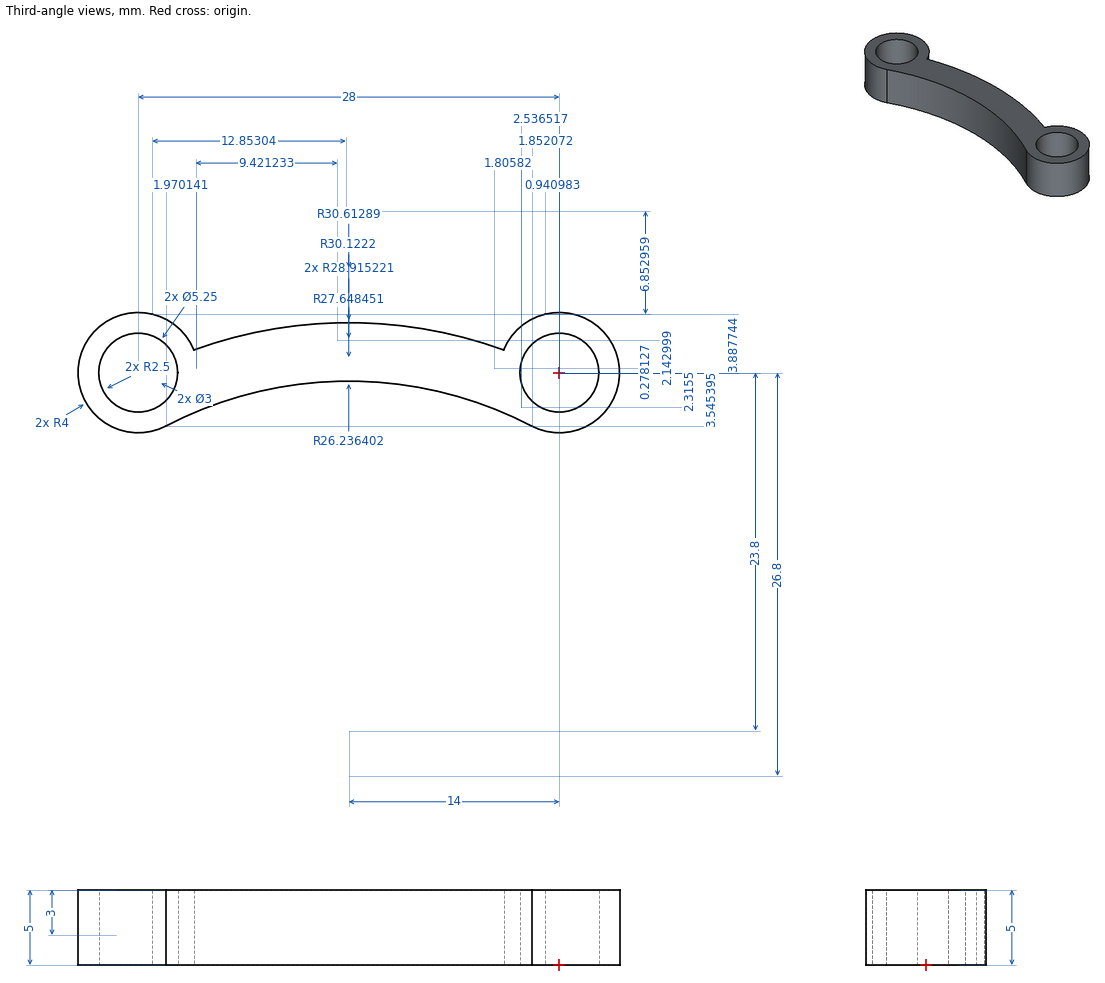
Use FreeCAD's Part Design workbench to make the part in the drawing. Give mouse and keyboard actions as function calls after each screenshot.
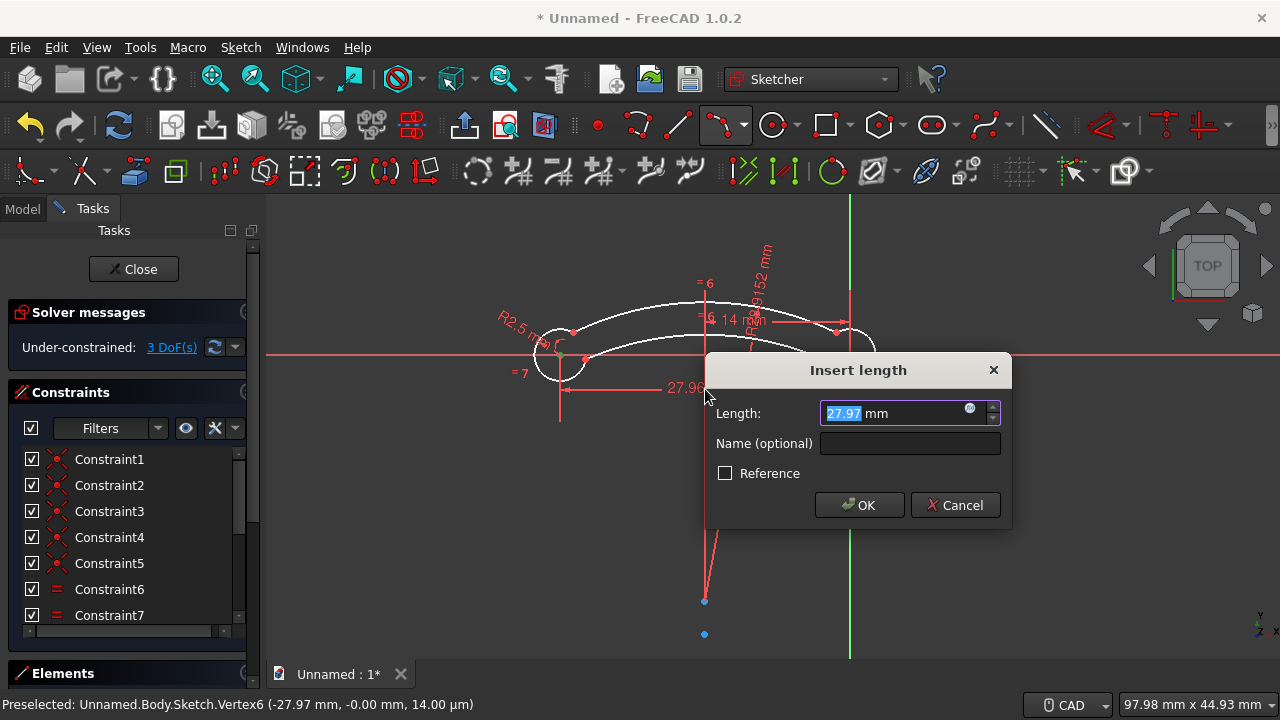
text(28)
key(Return)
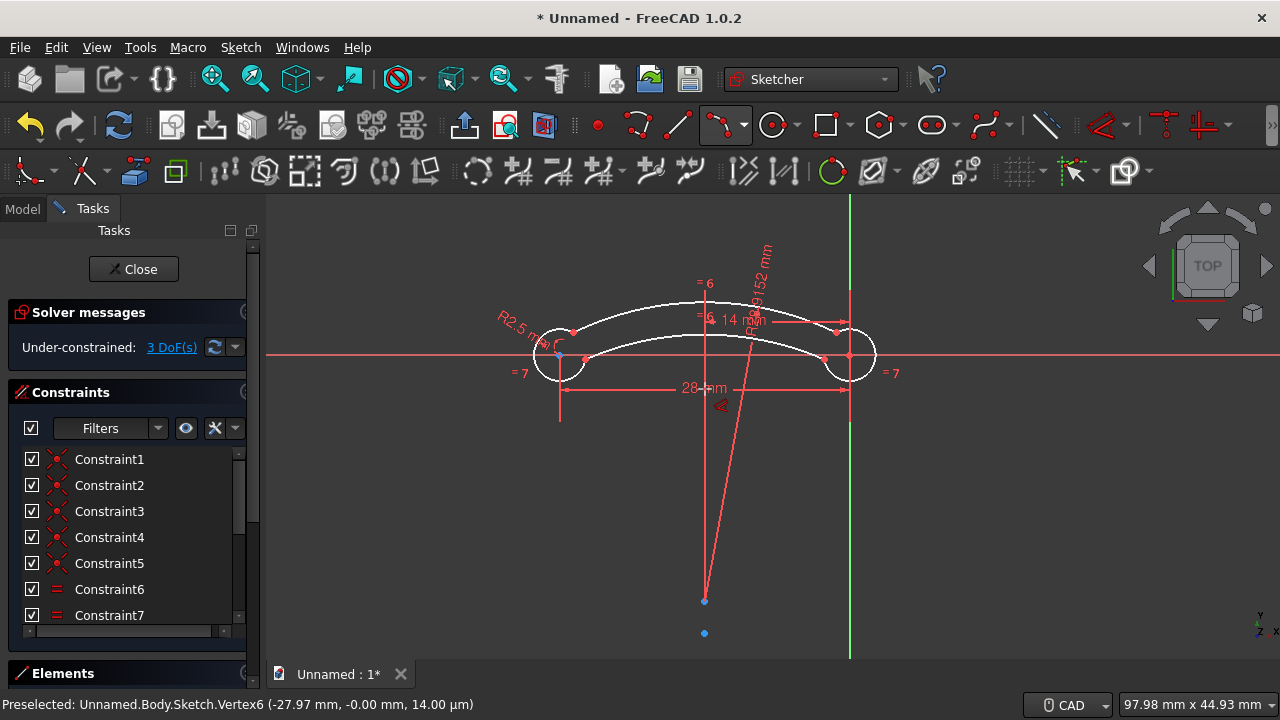
scroll(705, 222, up, 3)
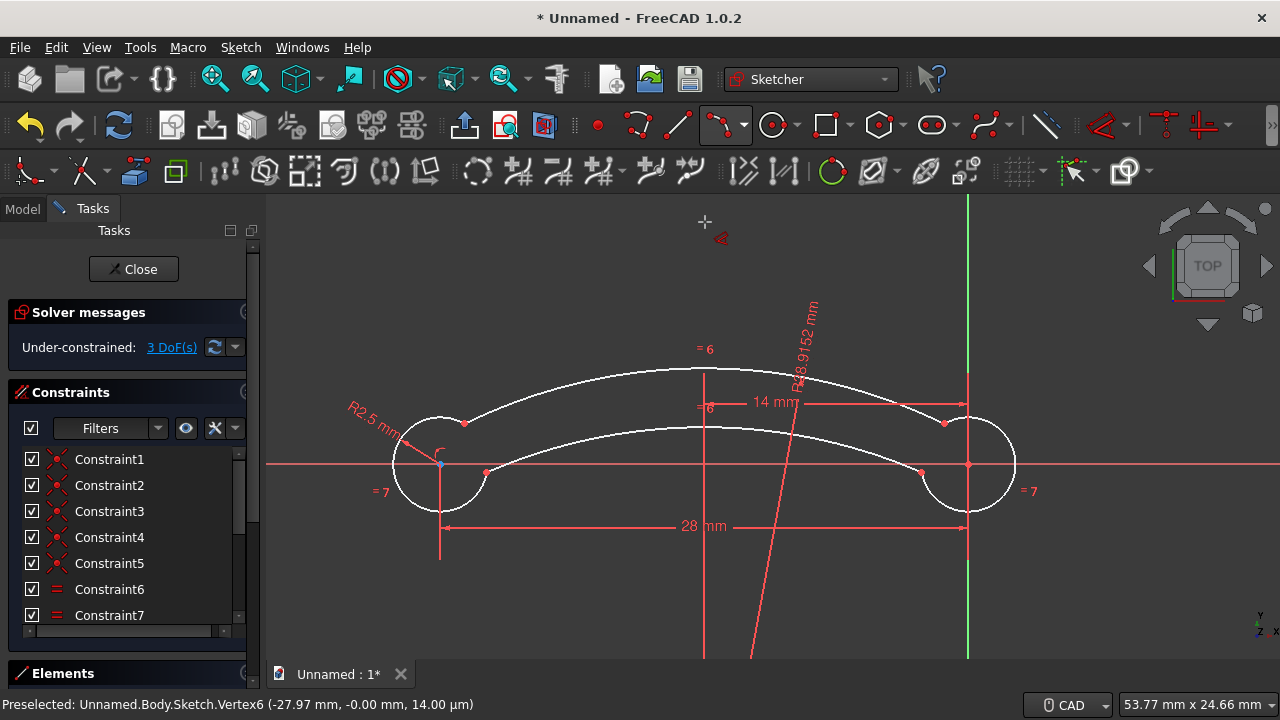
scroll(705, 228, down, 4)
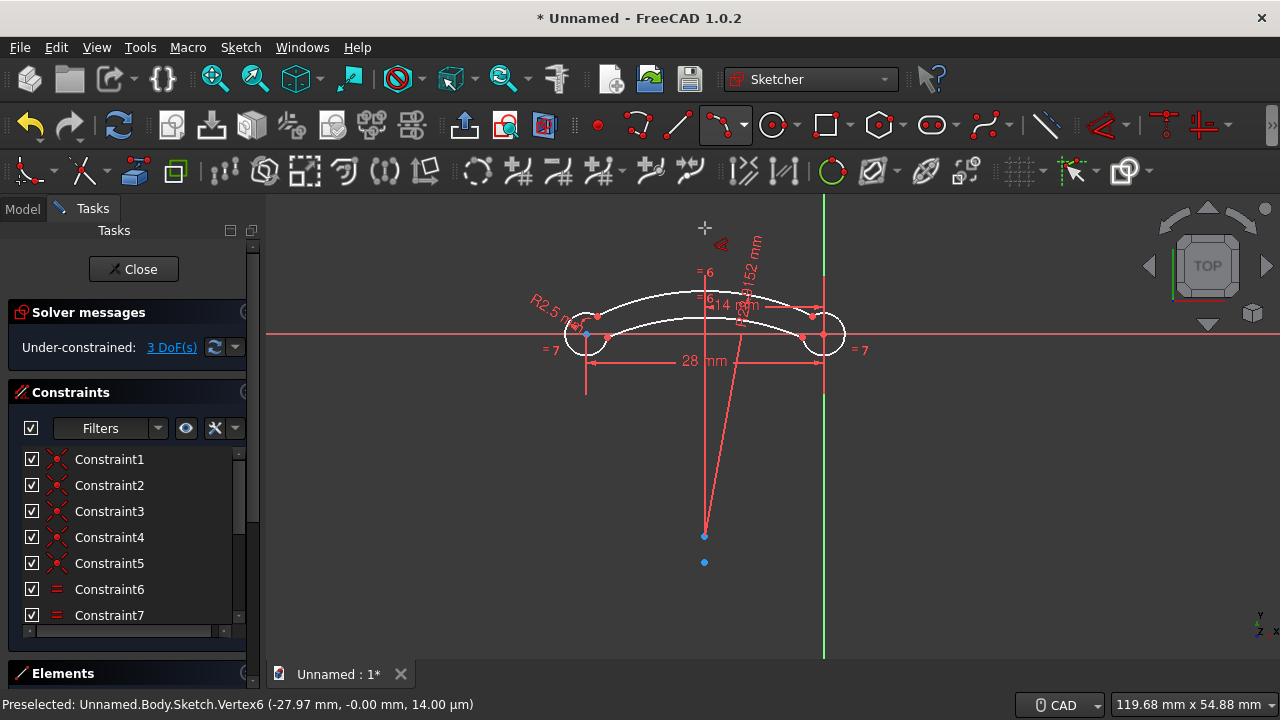
click(705, 563)
click(764, 597)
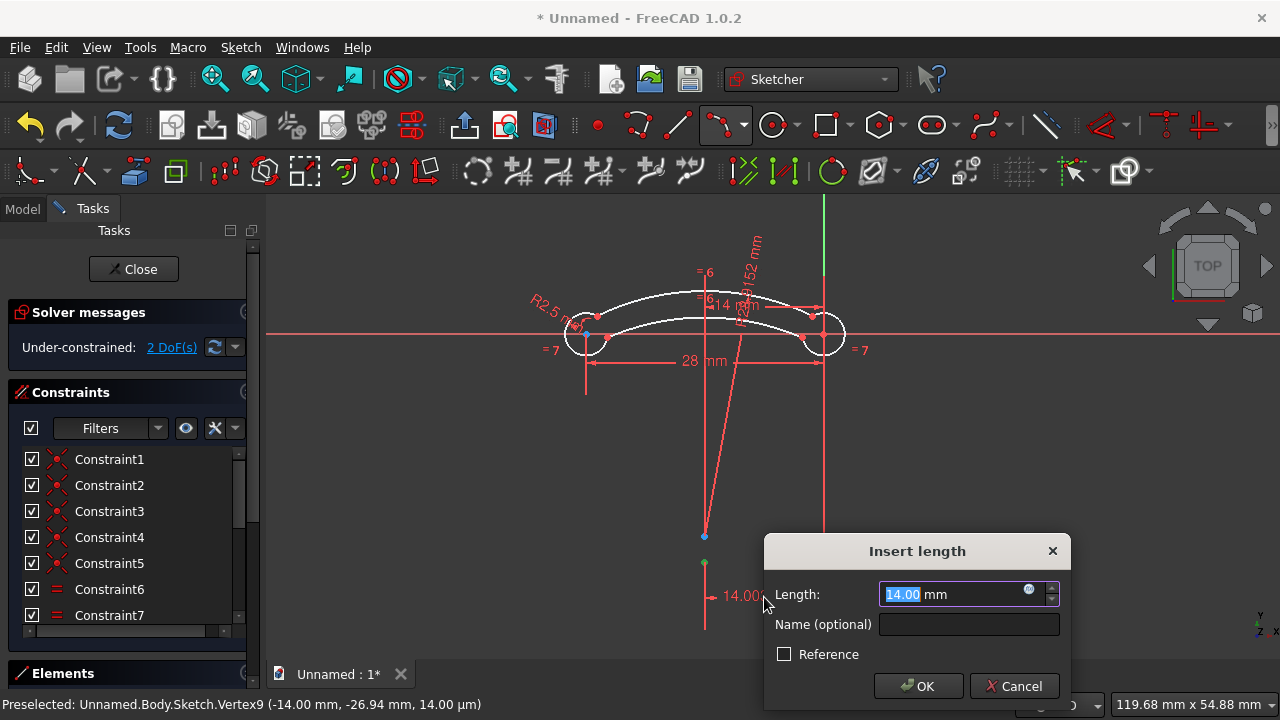
text(14)
key(Return)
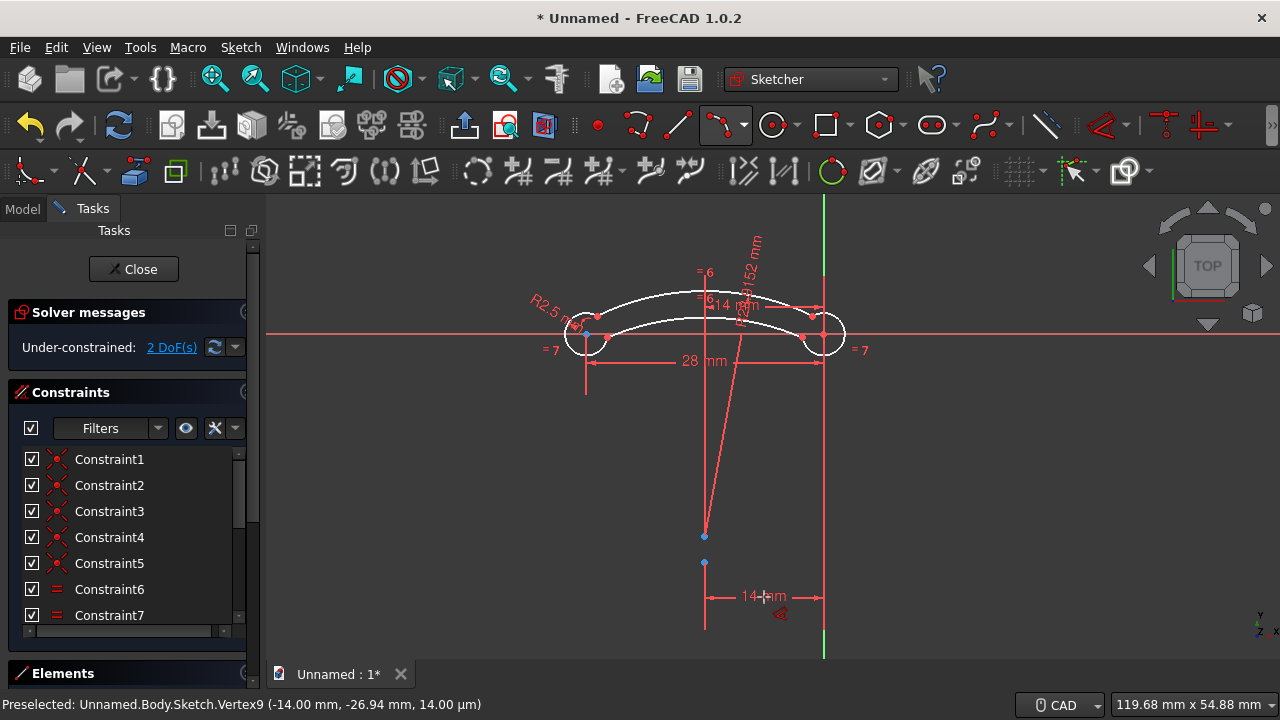
click(705, 536)
click(858, 435)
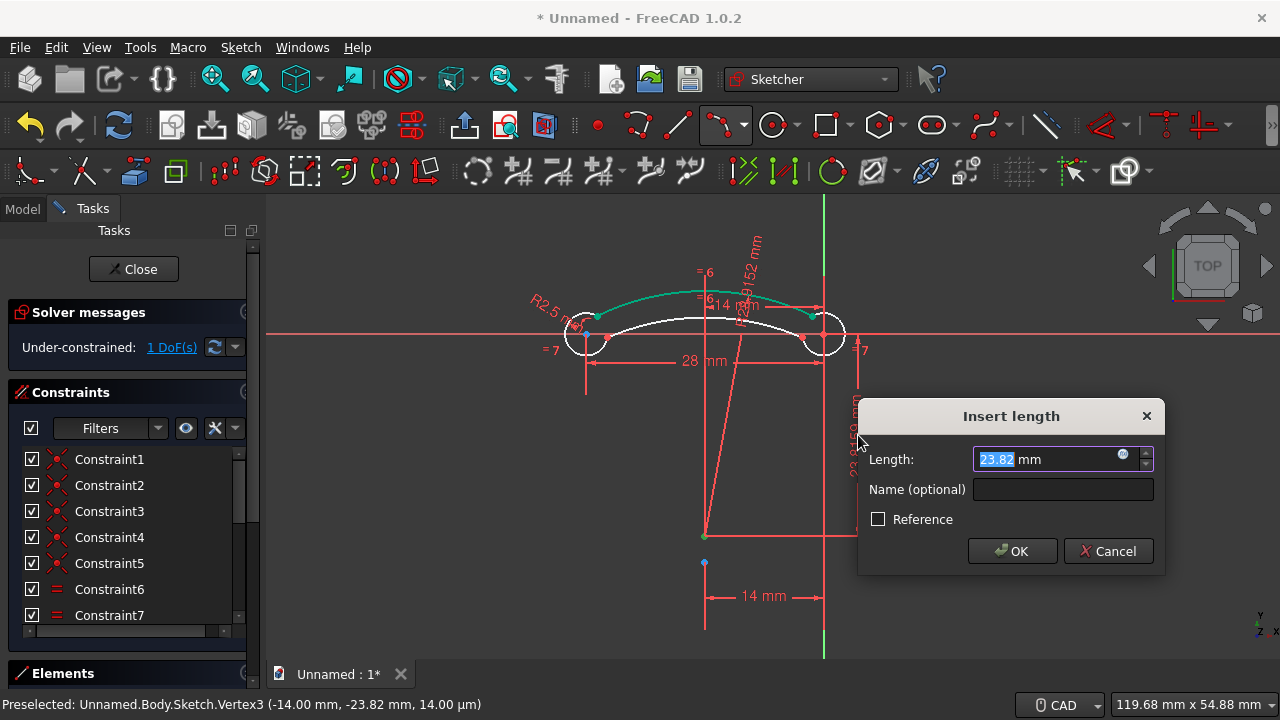
text(23.8)
key(Return)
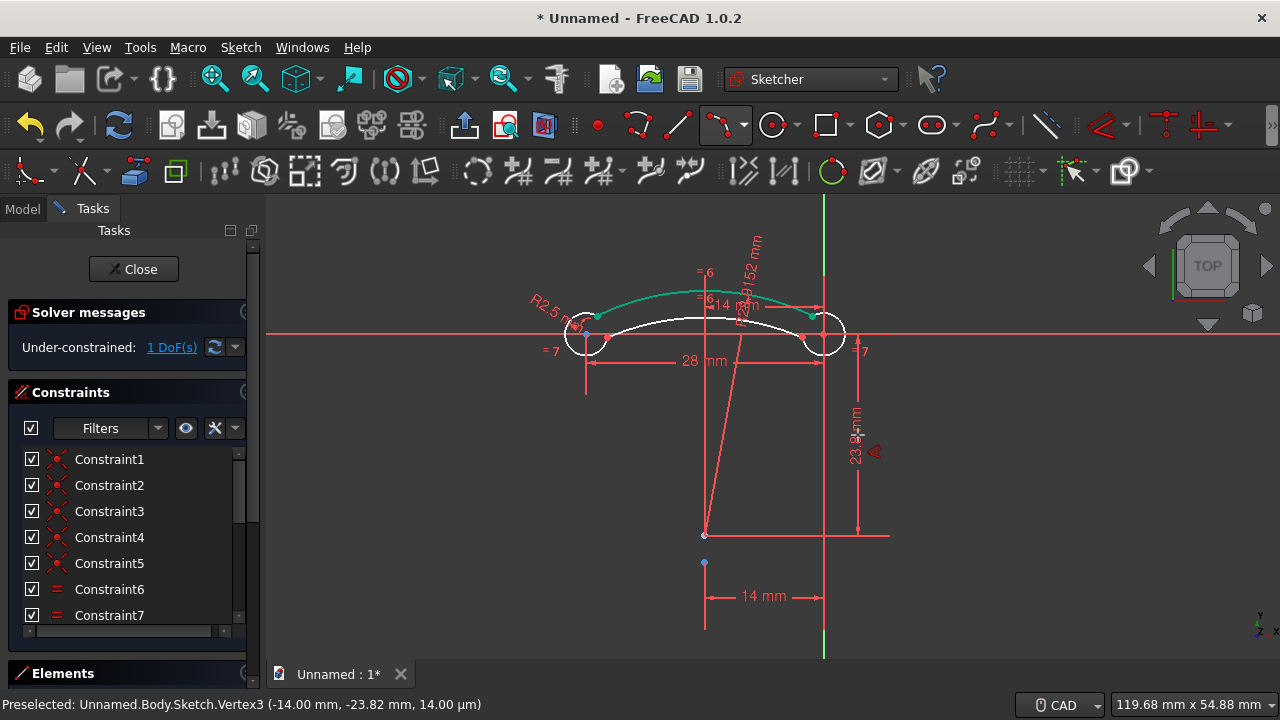
click(705, 563)
click(858, 396)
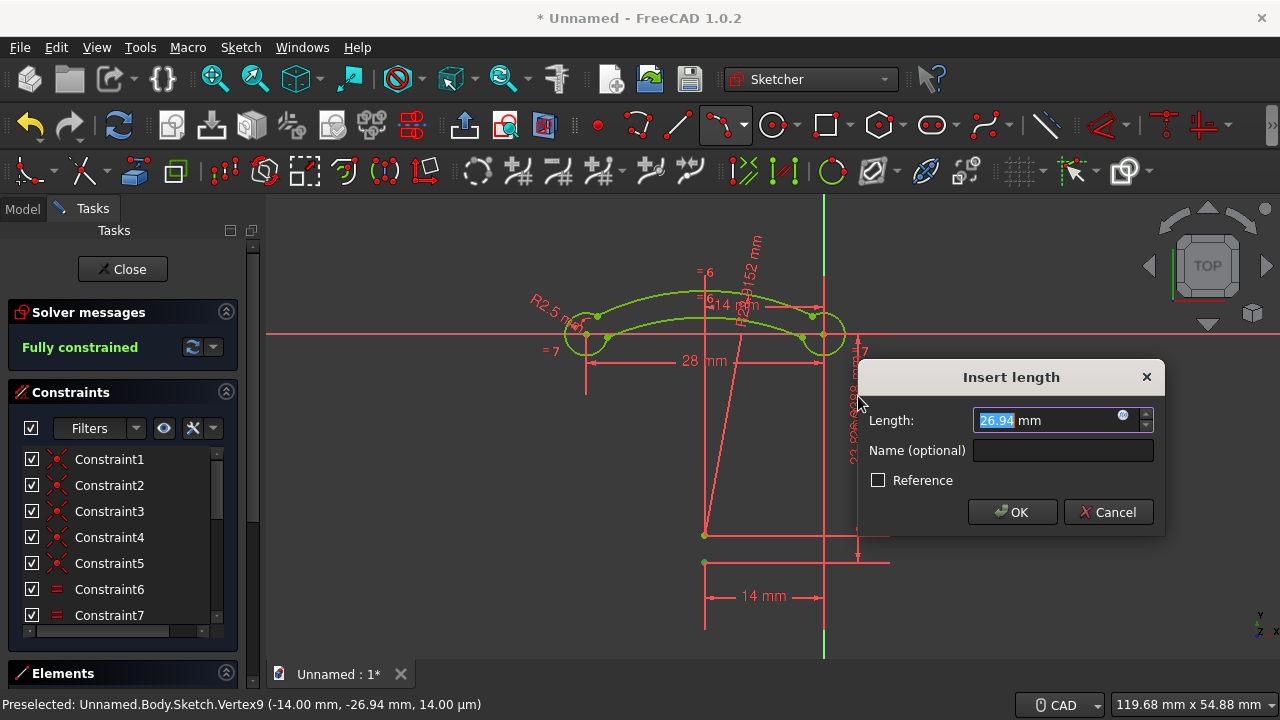
text(26.8)
key(Return)
key(Escape)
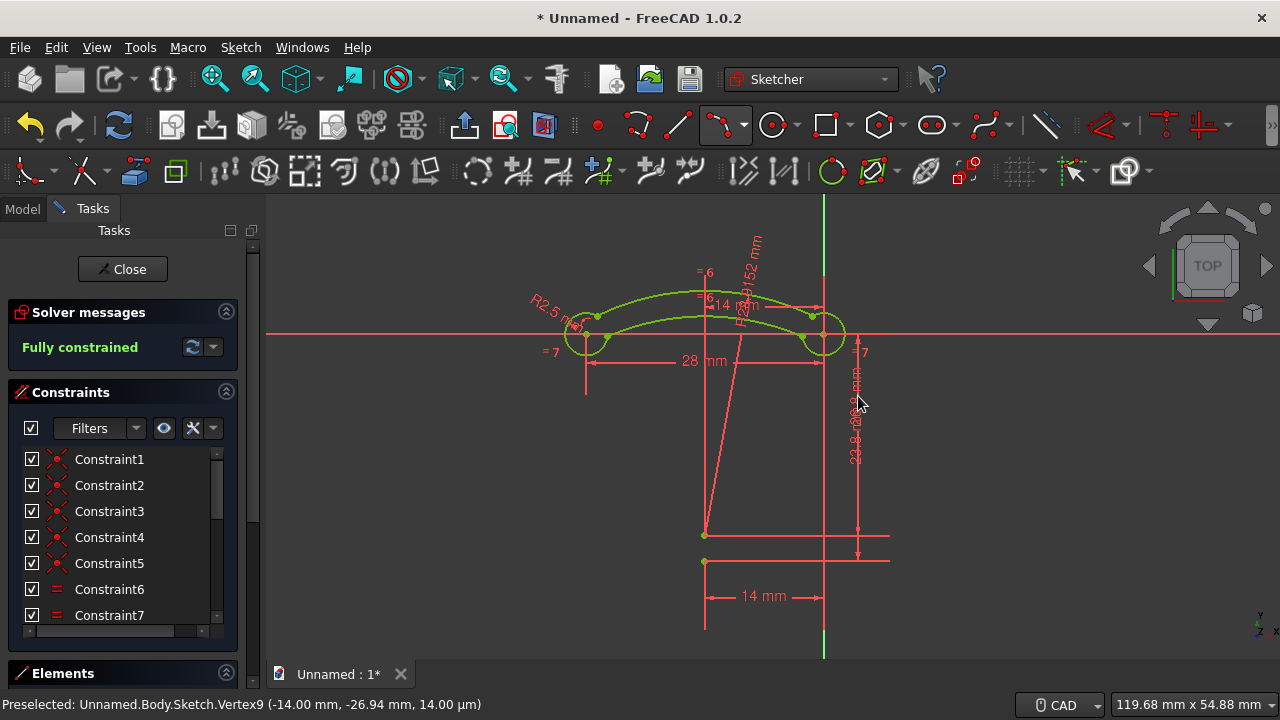
click(123, 269)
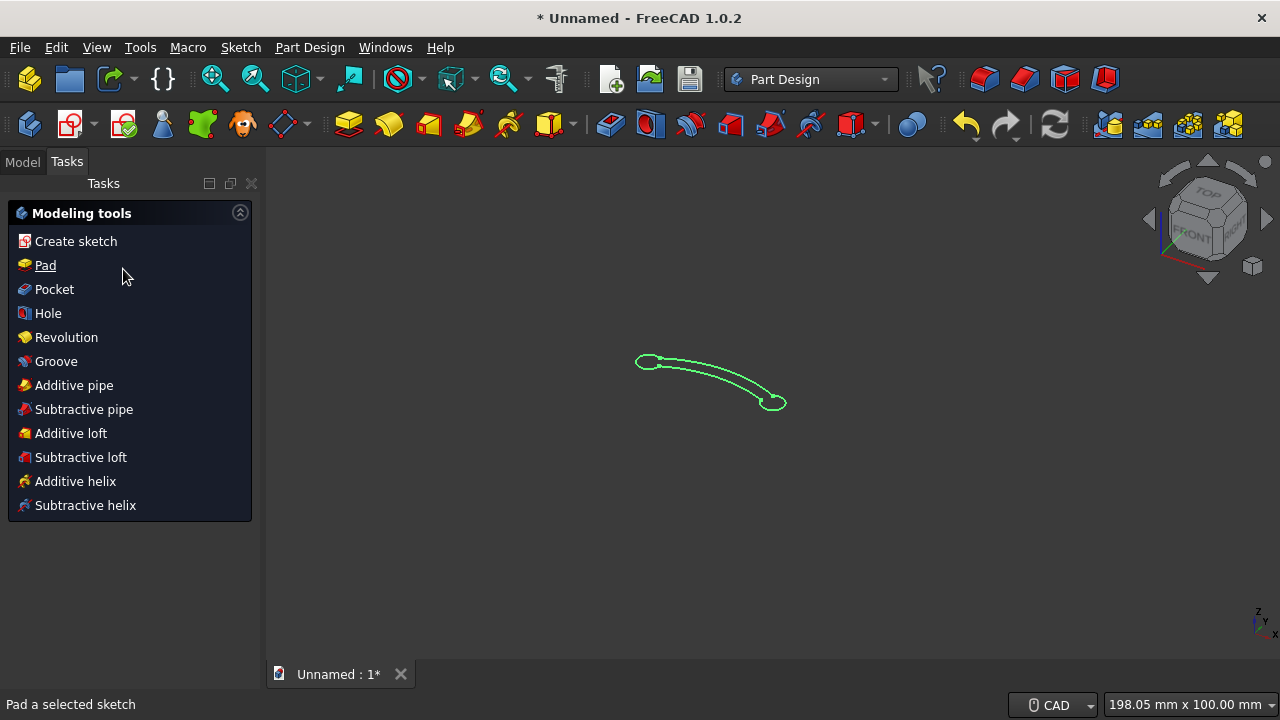
click(350, 124)